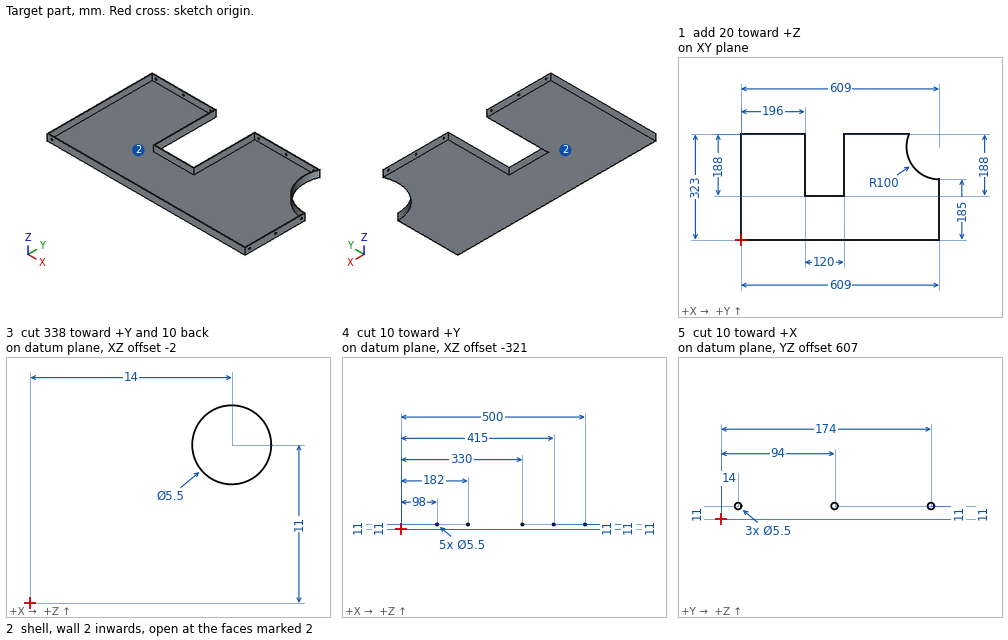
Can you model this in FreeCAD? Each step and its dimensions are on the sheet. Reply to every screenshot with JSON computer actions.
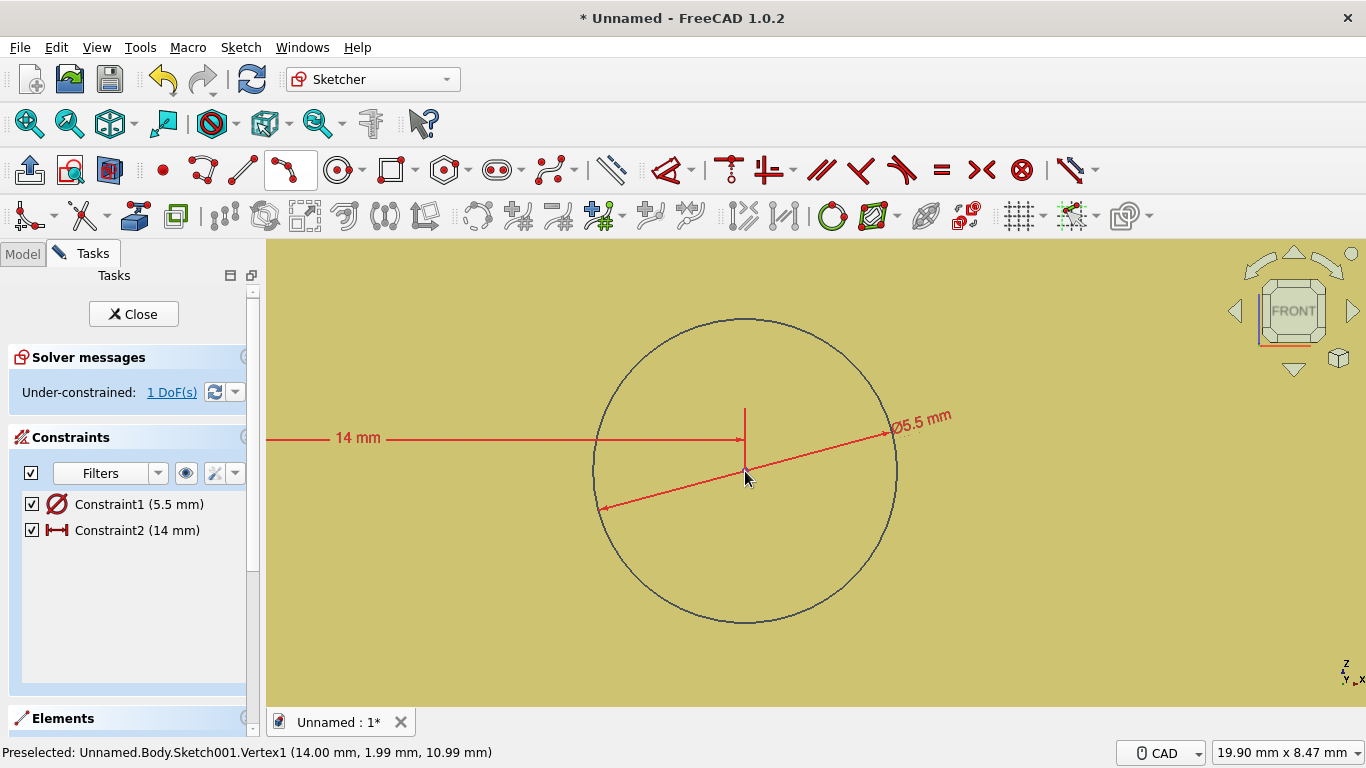
{"action": "left_click", "coordinate": [745, 471]}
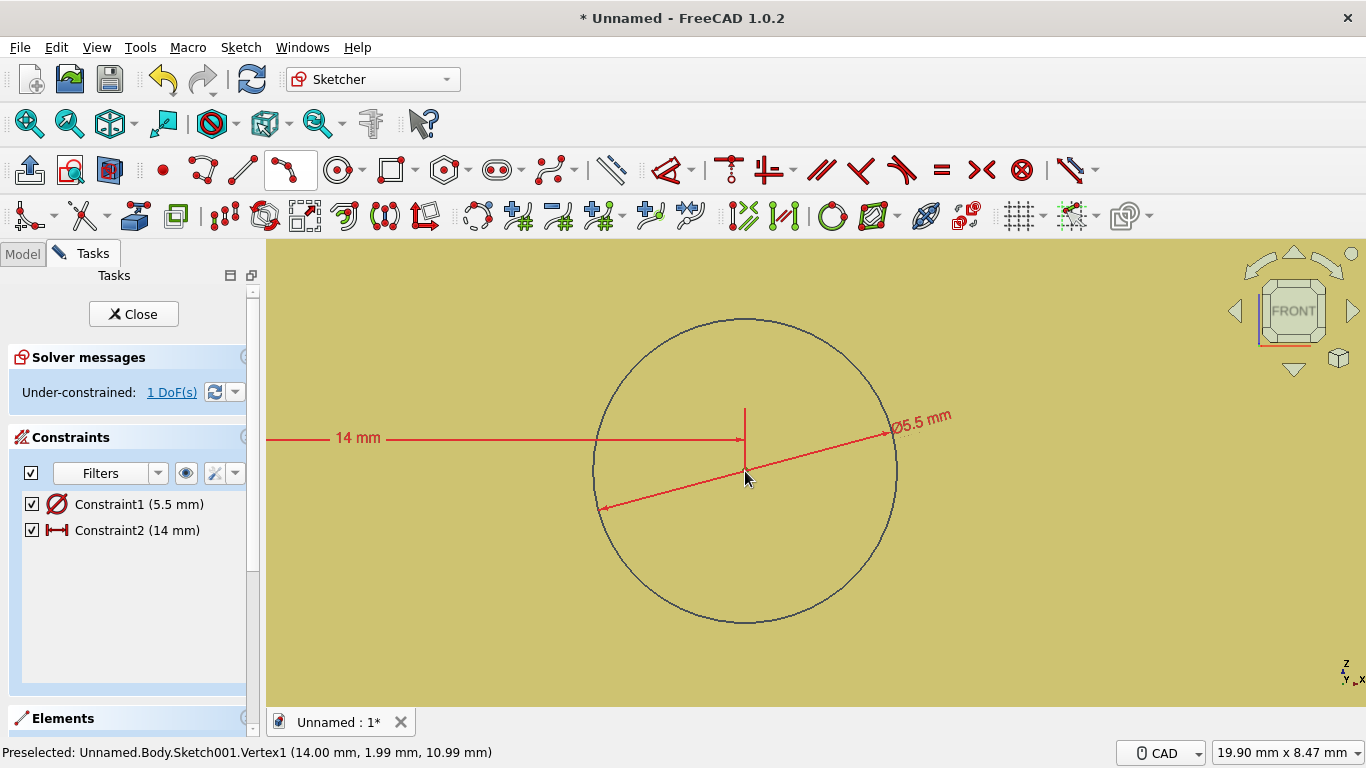
{"action": "key", "text": "i"}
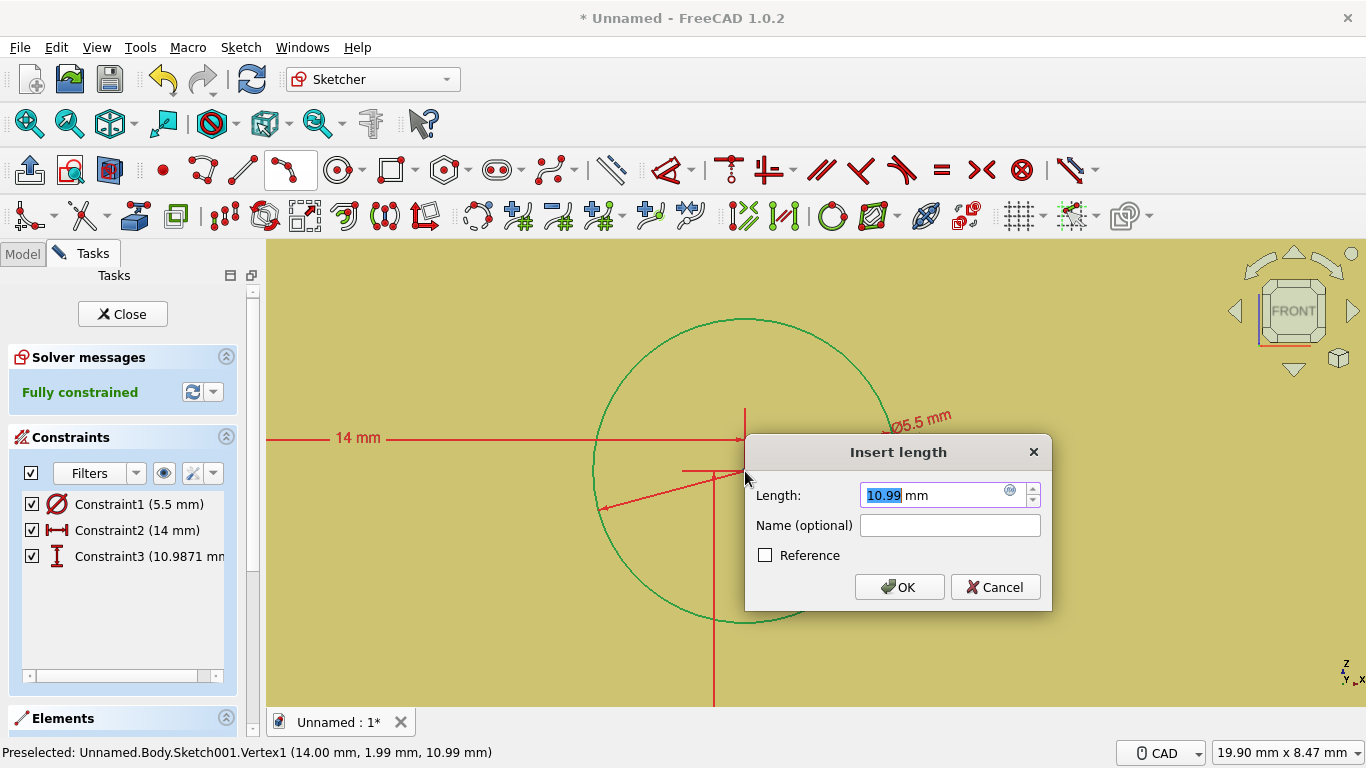
{"action": "type", "text": "11"}
{"action": "key", "text": "Return"}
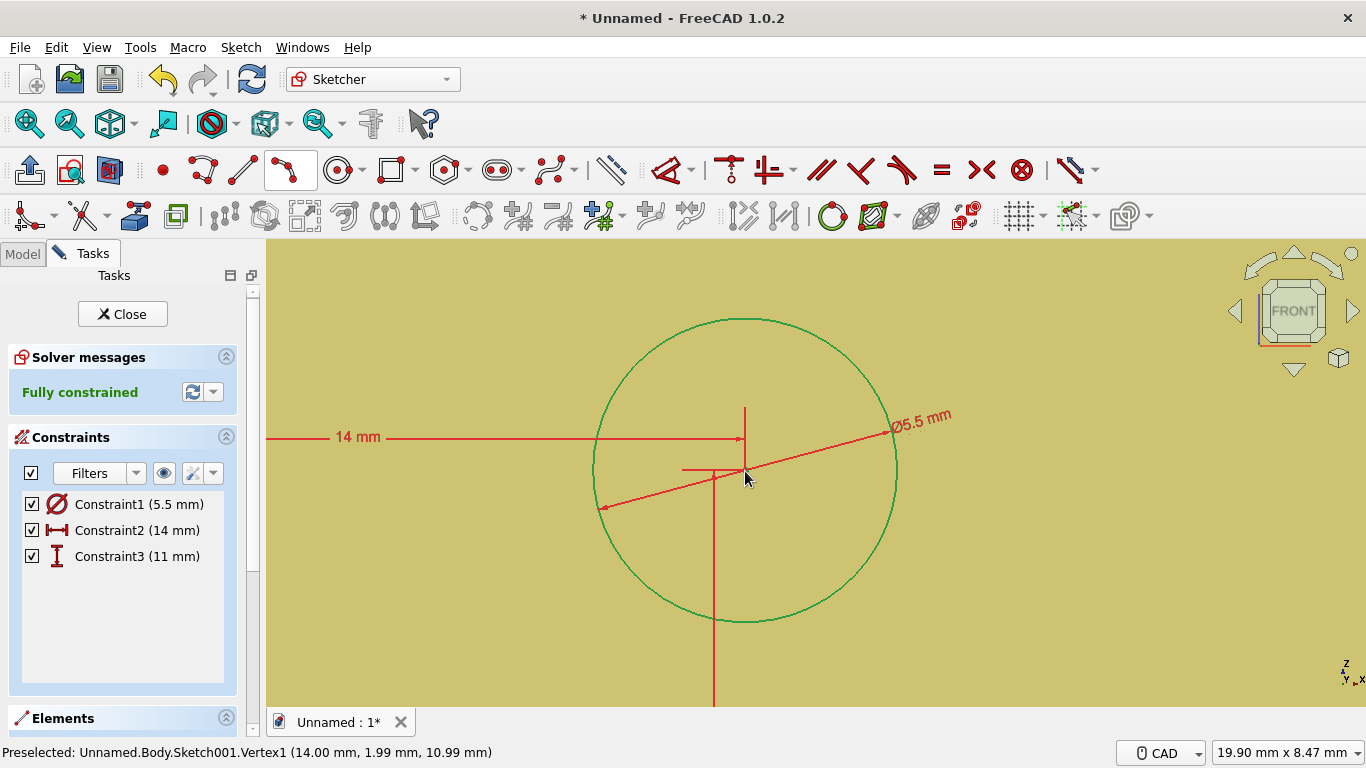
{"action": "left_click", "coordinate": [123, 314]}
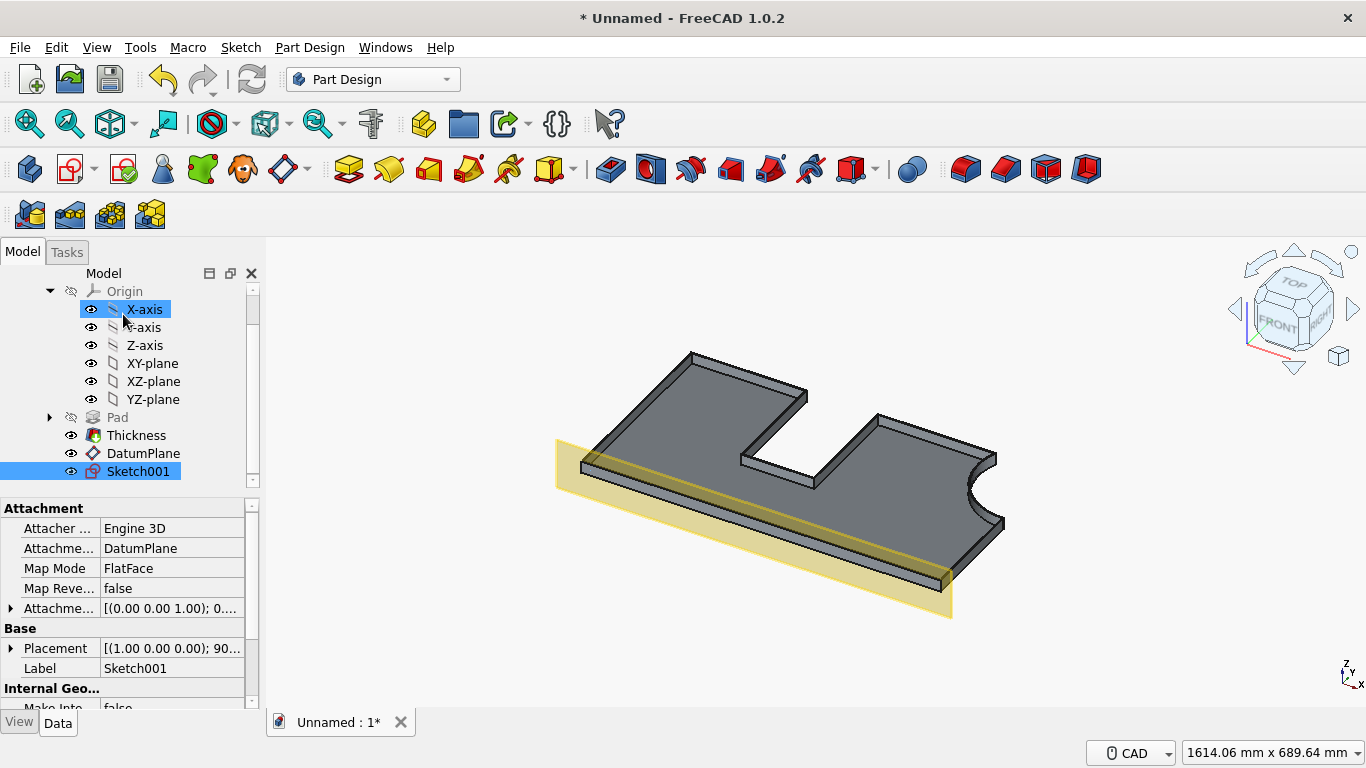
{"action": "left_click", "coordinate": [612, 170]}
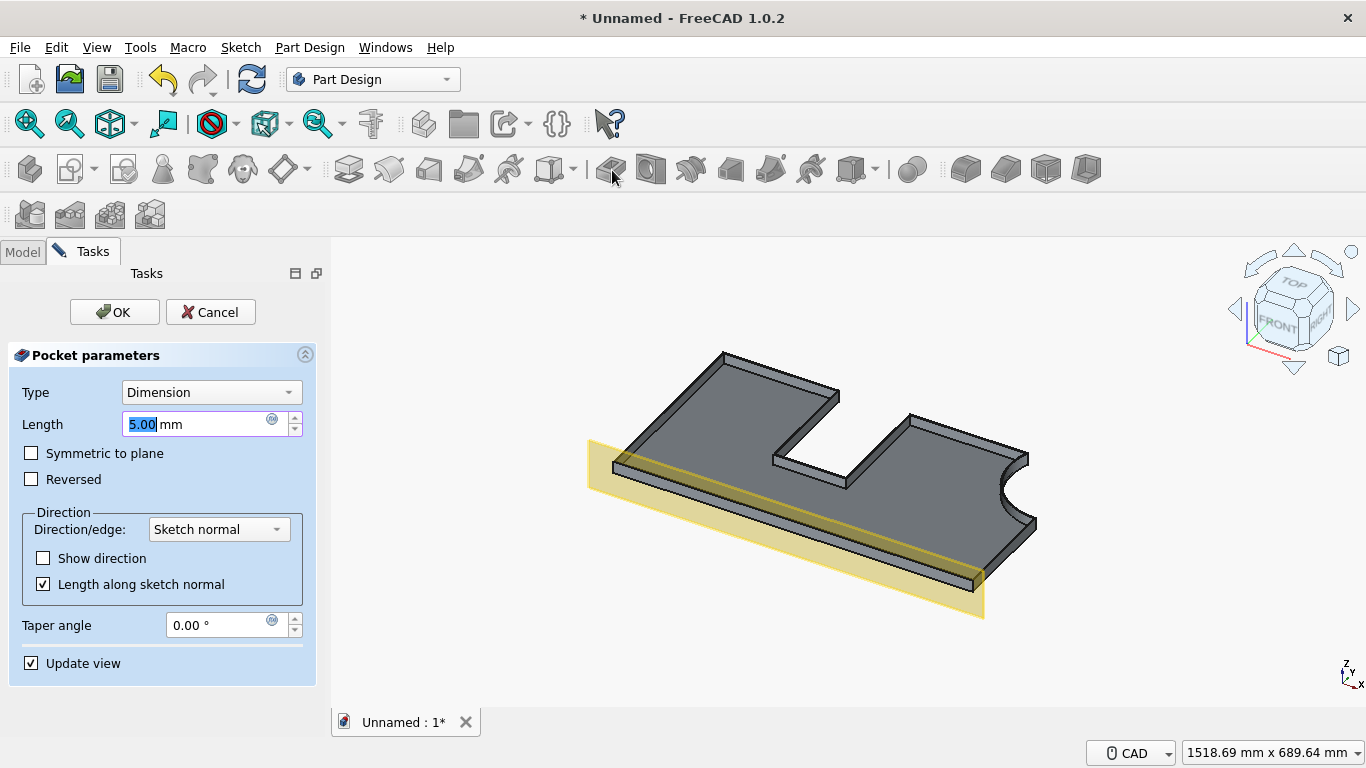
{"action": "left_click", "coordinate": [212, 392]}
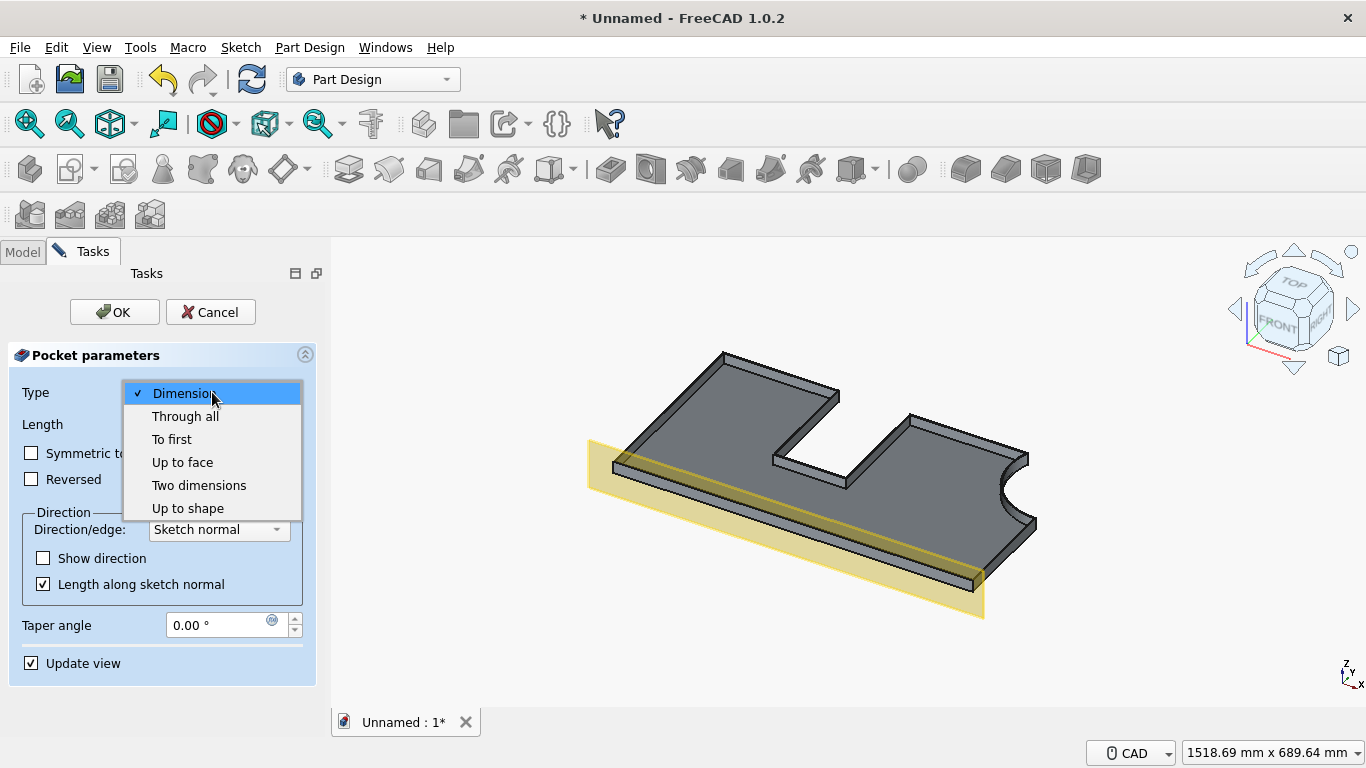
{"action": "left_click", "coordinate": [212, 486]}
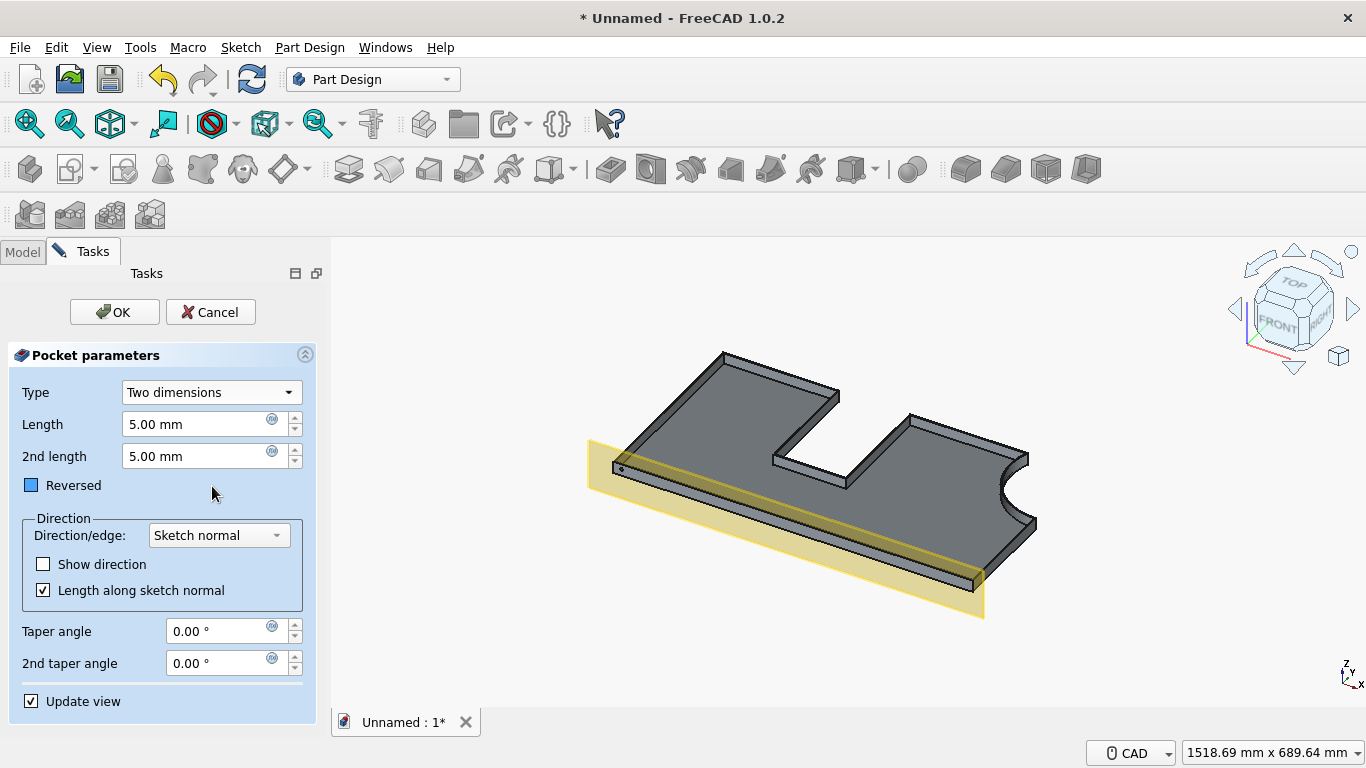
{"action": "triple_click", "coordinate": [204, 424]}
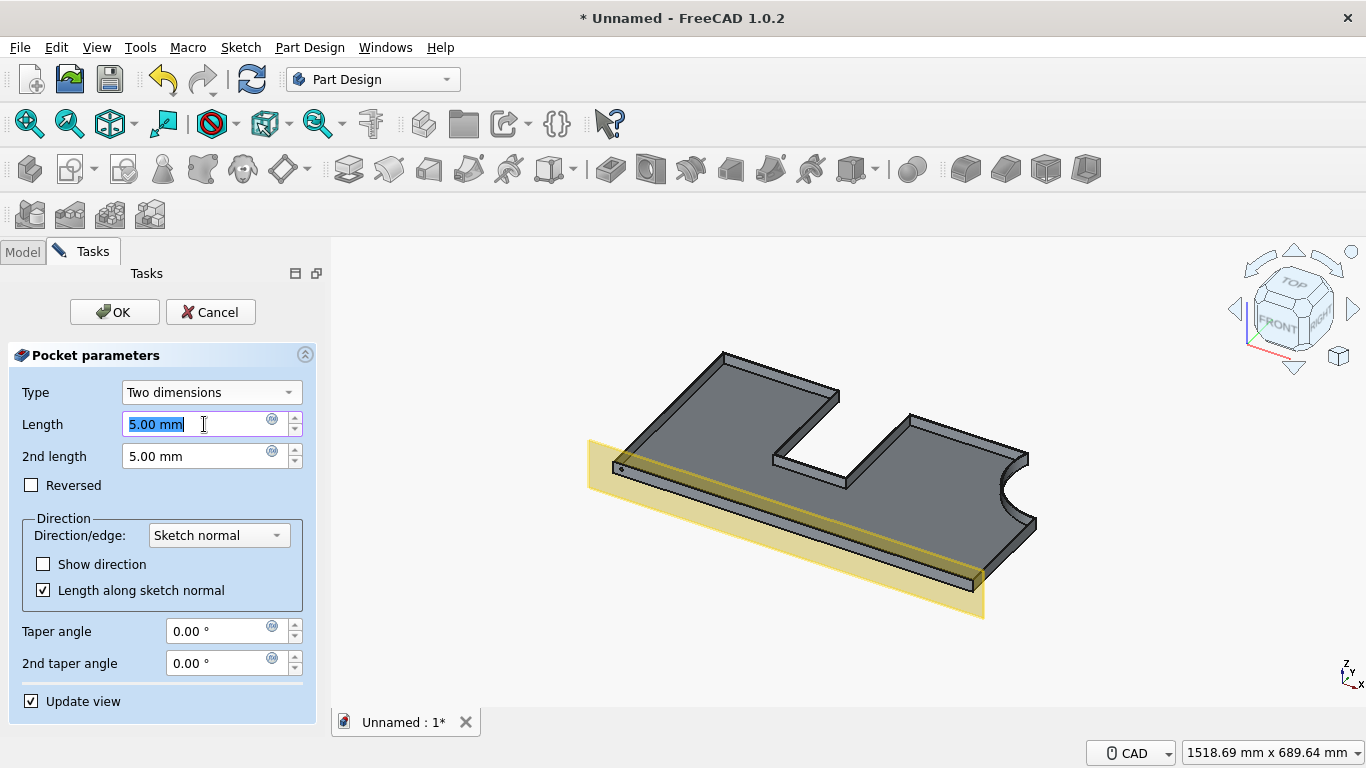
{"action": "type", "text": "338"}
{"action": "key", "text": "Tab"}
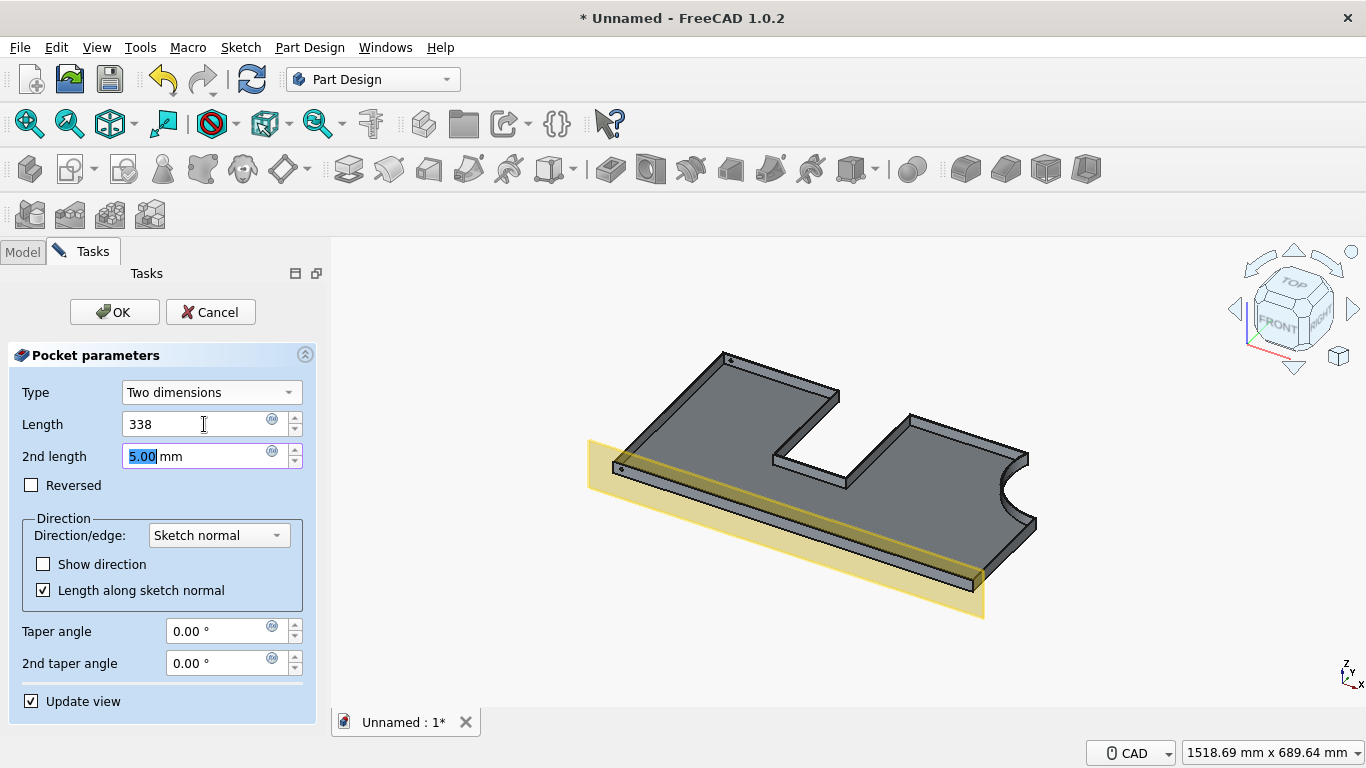
{"action": "type", "text": "10"}
{"action": "key", "text": "Tab"}